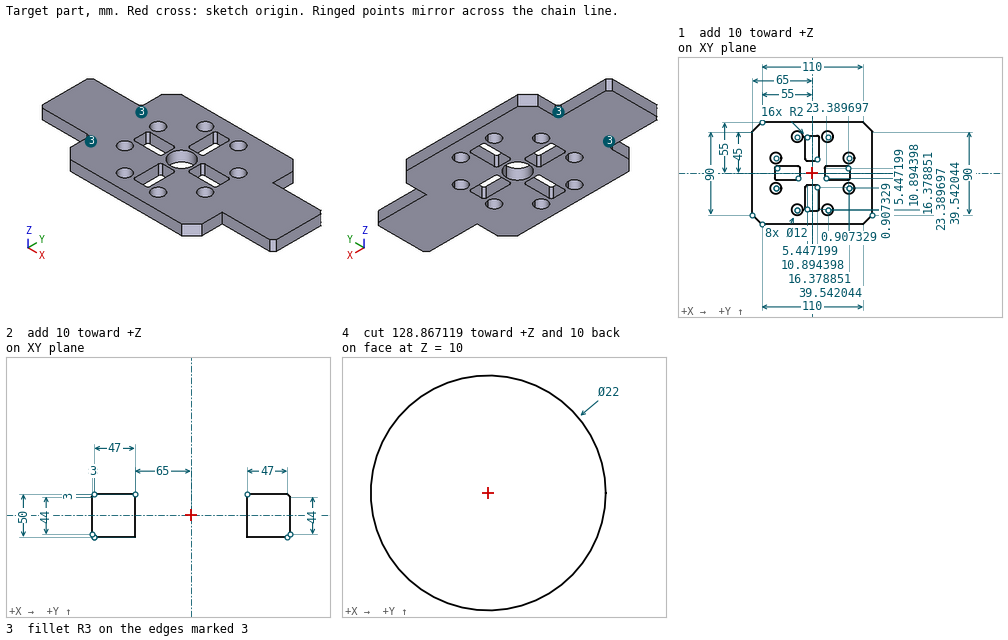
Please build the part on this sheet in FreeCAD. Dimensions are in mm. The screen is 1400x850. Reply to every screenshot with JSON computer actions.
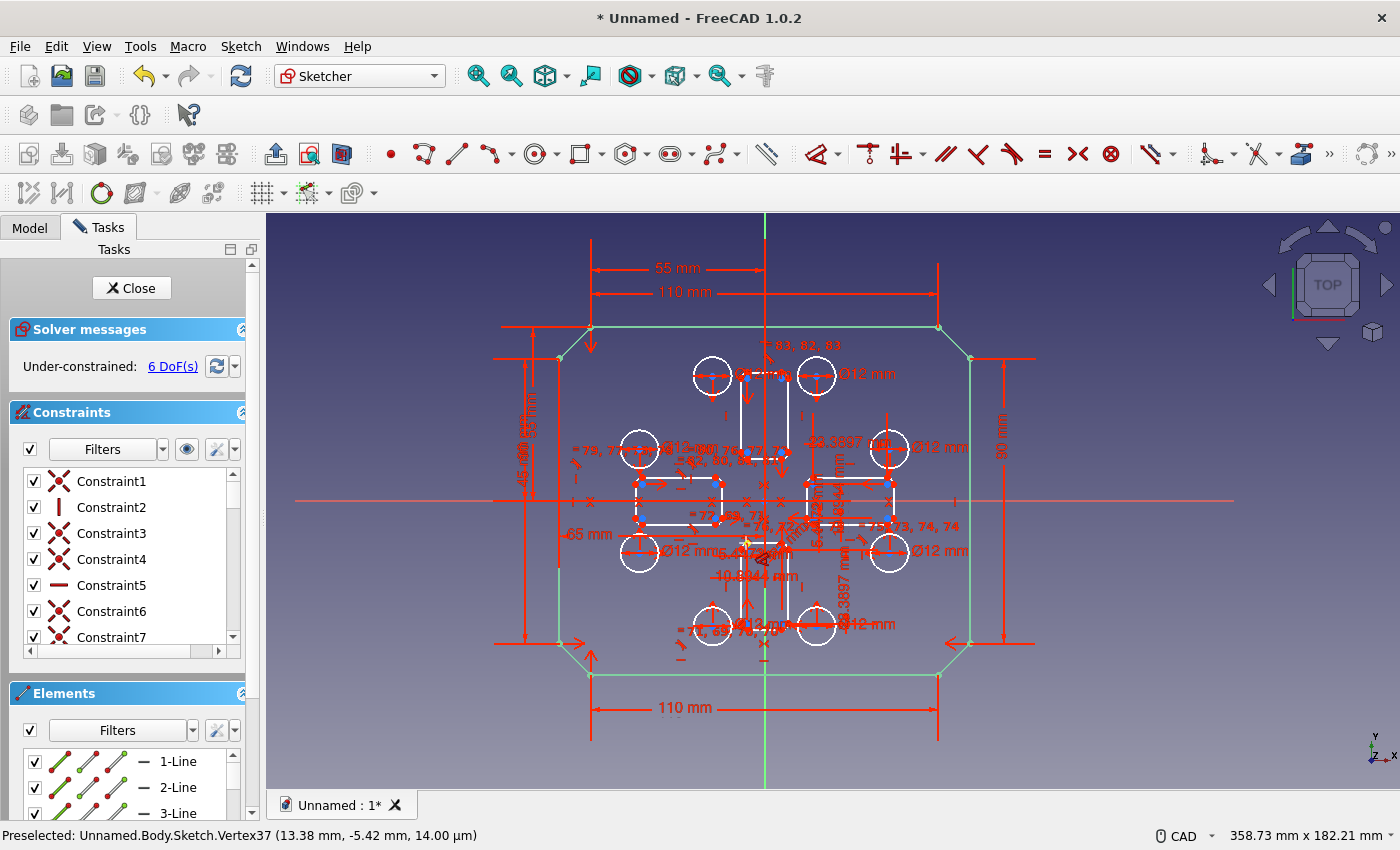
{"action": "left_click", "coordinate": [817, 626]}
{"action": "left_click", "coordinate": [791, 660]}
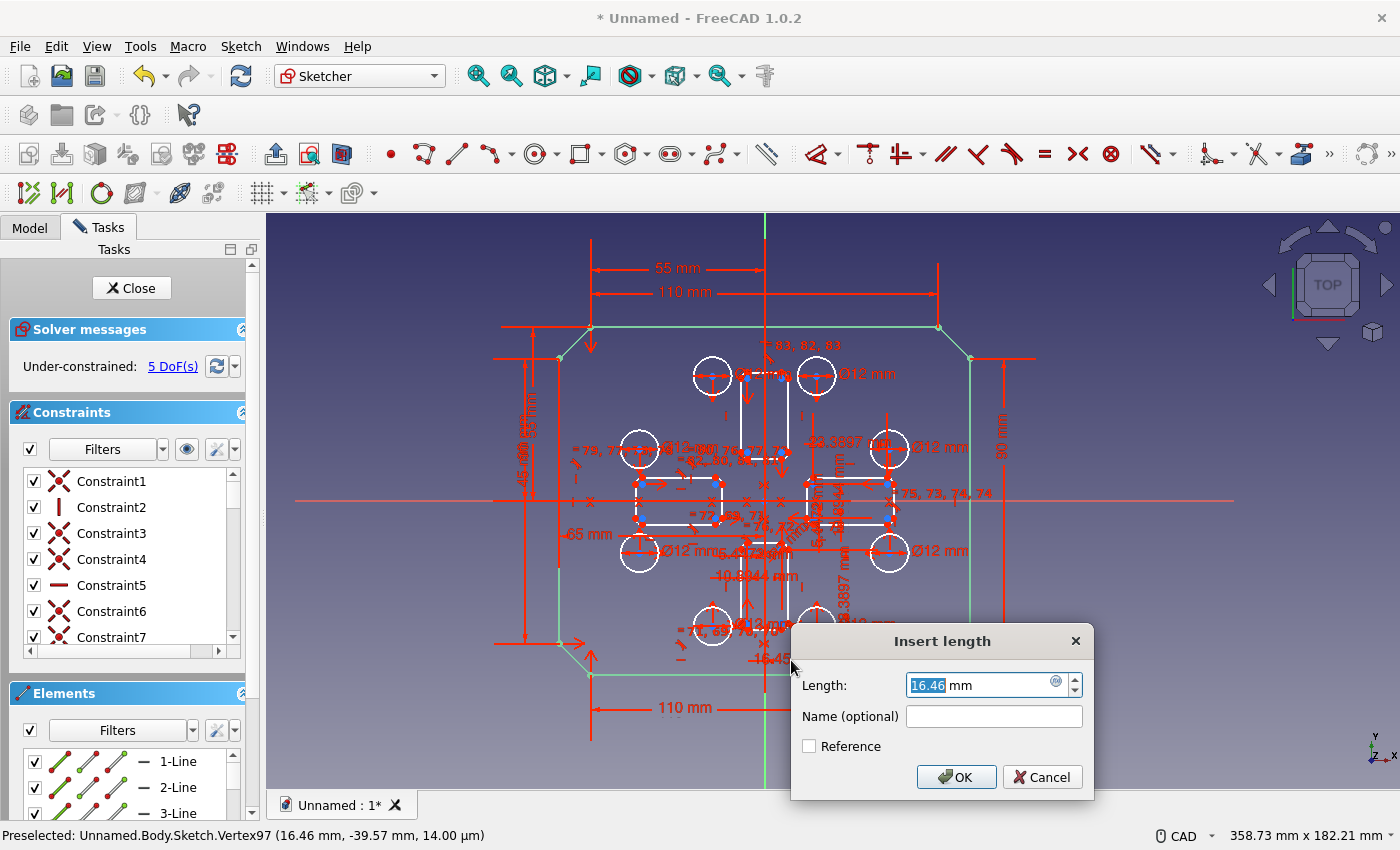
{"action": "type", "text": "16.378851"}
{"action": "key", "text": "Return"}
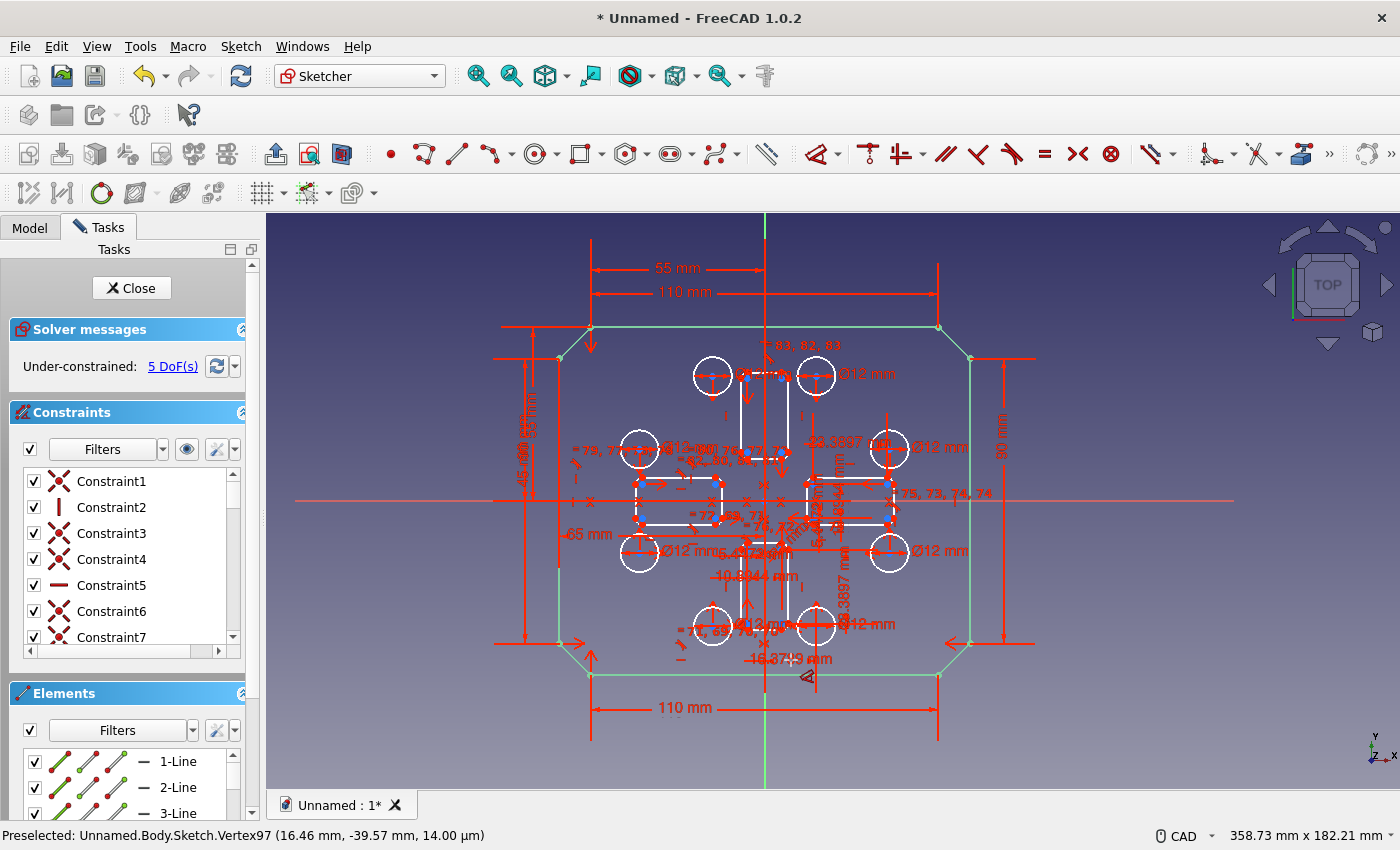
{"action": "left_click", "coordinate": [816, 626]}
{"action": "left_click", "coordinate": [850, 564]}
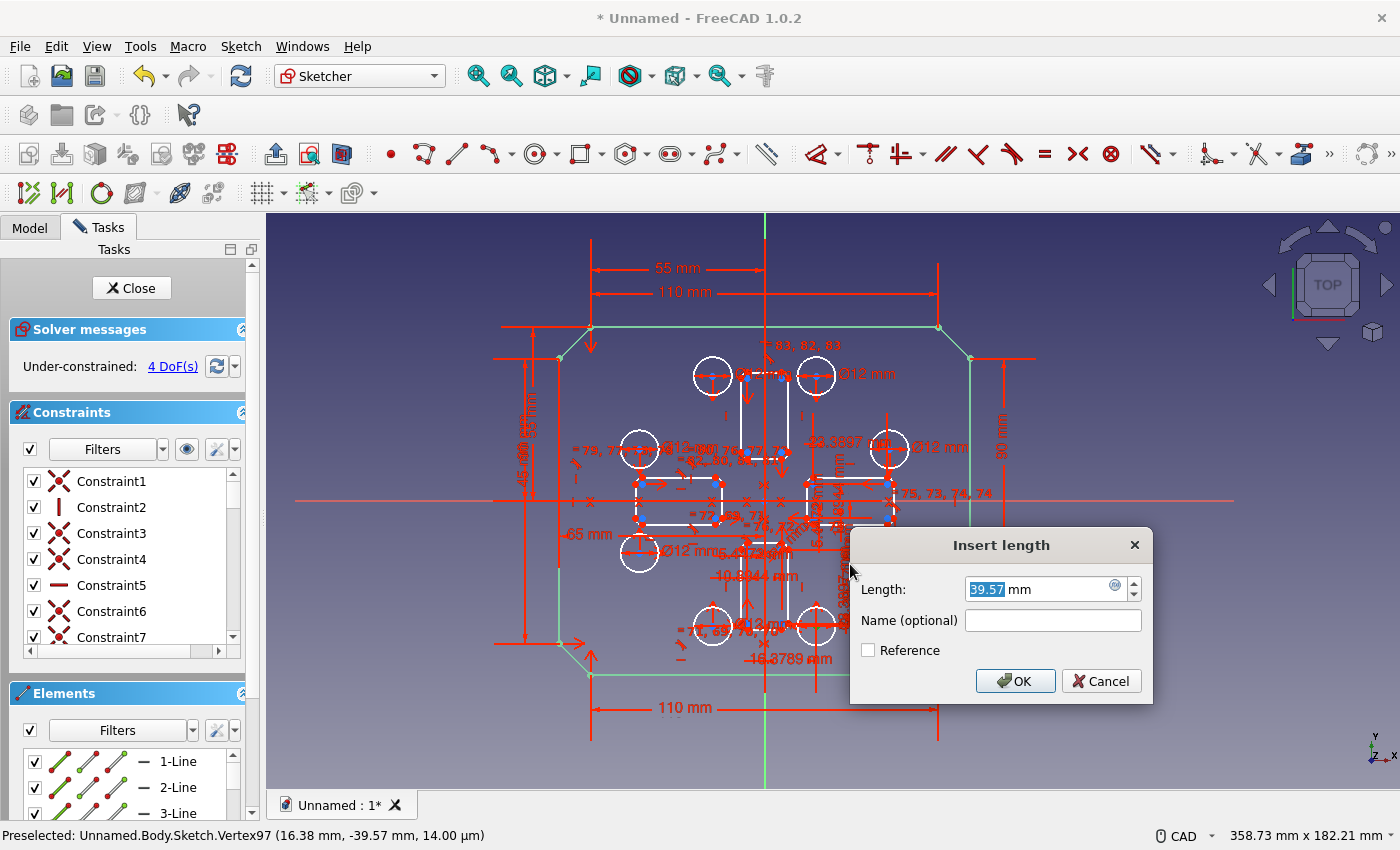
{"action": "type", "text": "39.542044"}
{"action": "key", "text": "Return"}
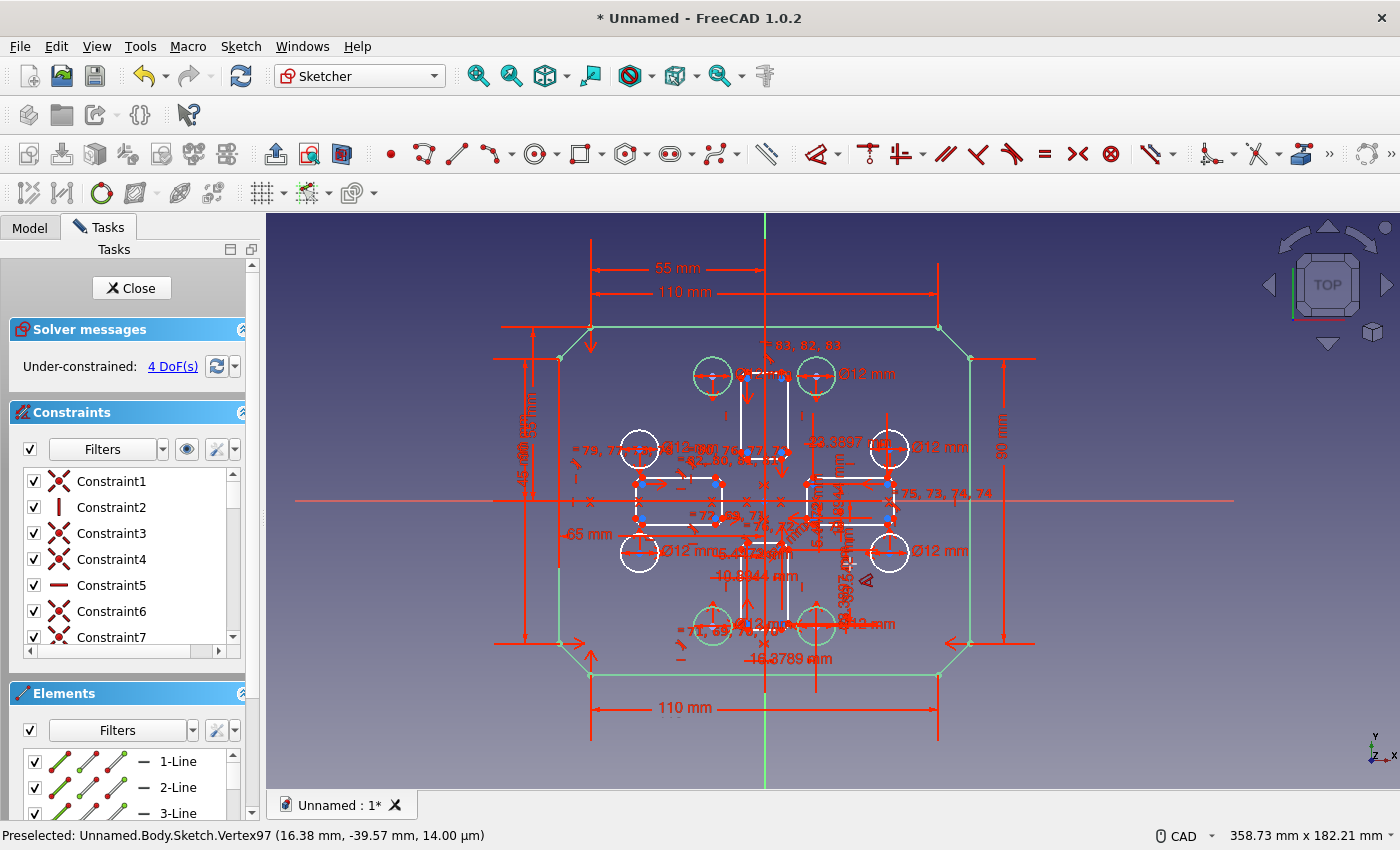
{"action": "left_click", "coordinate": [890, 553]}
{"action": "left_click", "coordinate": [798, 467]}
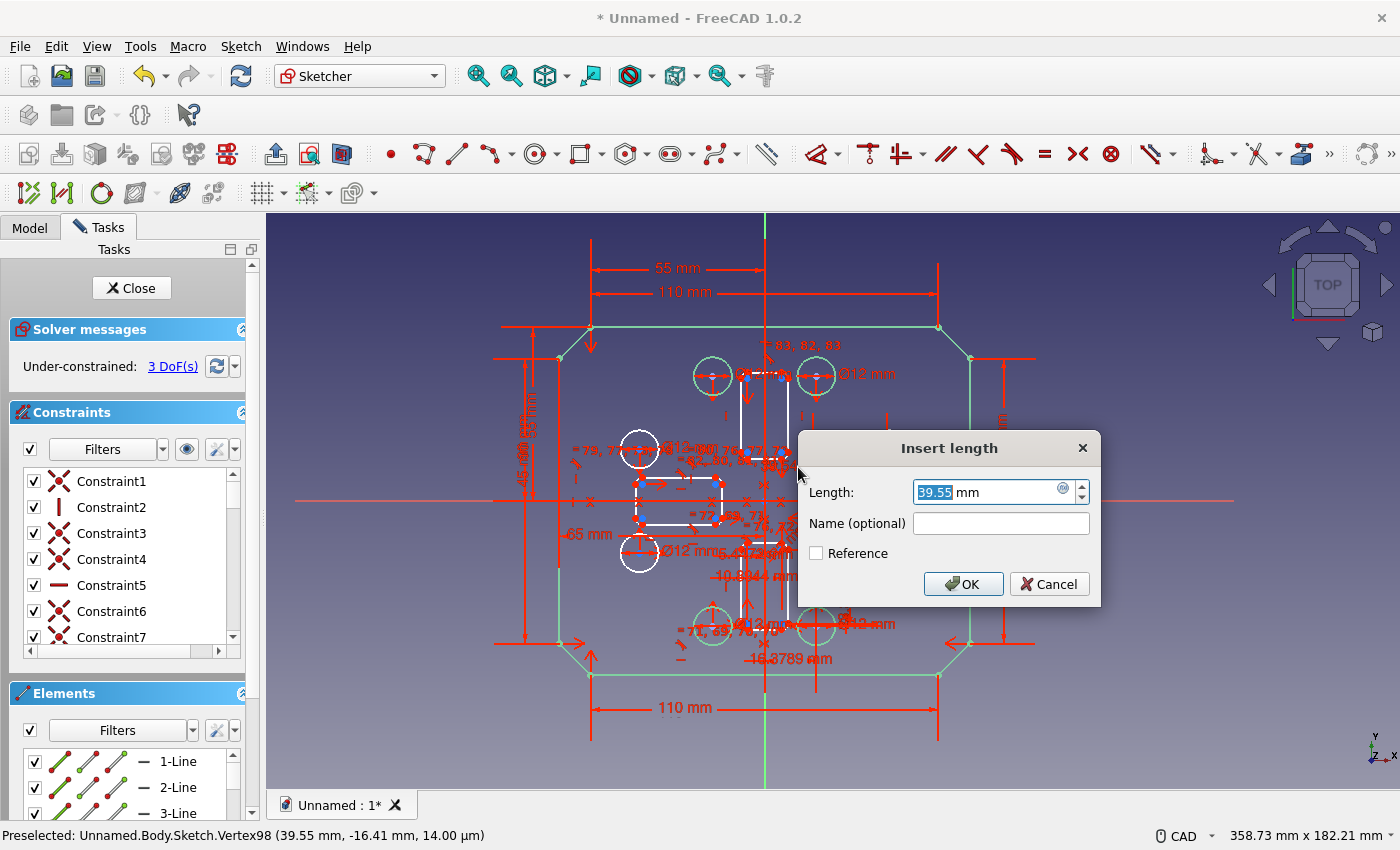
{"action": "type", "text": "39.542044"}
{"action": "key", "text": "Return"}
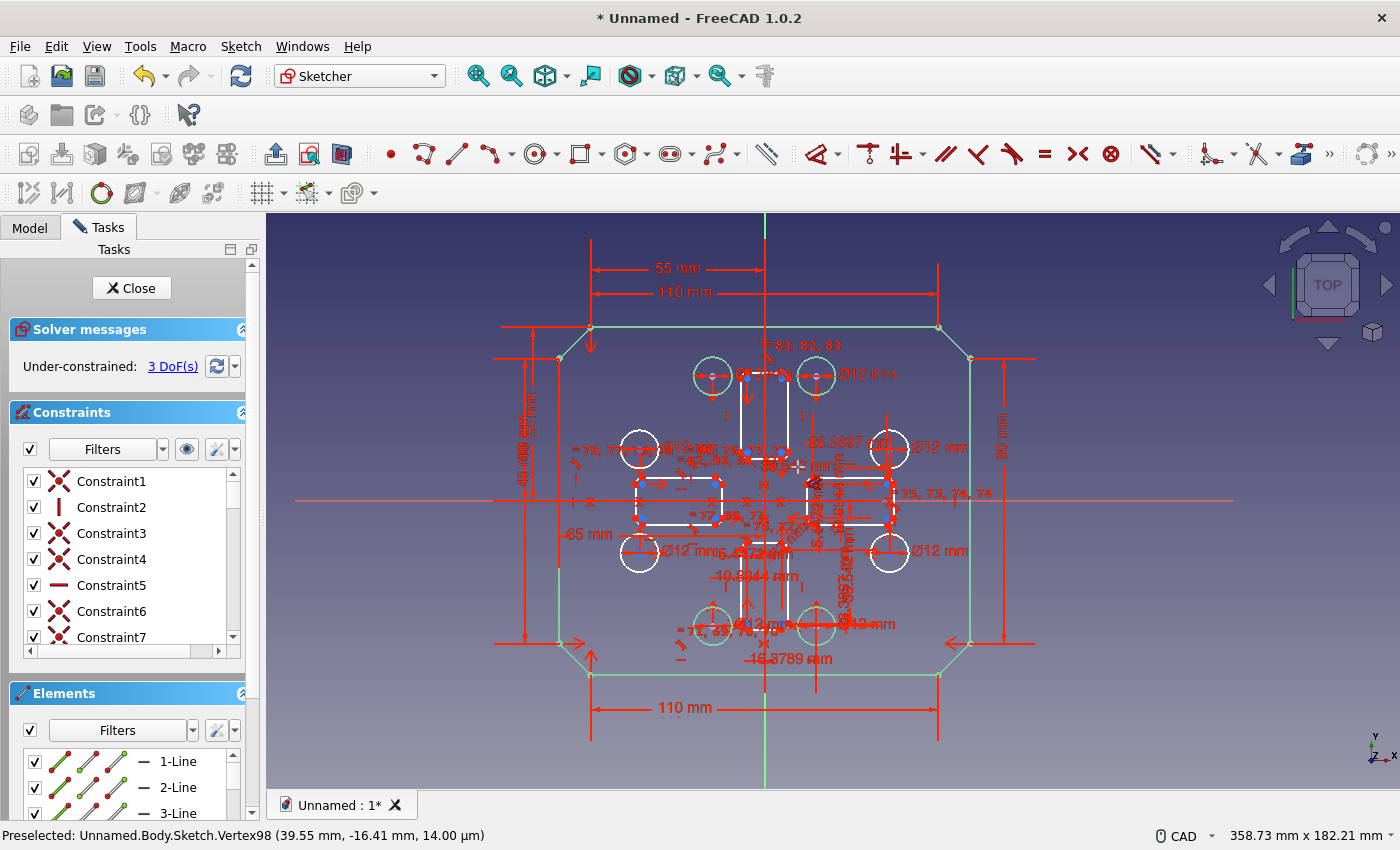
{"action": "left_click", "coordinate": [890, 553]}
{"action": "left_click", "coordinate": [924, 527]}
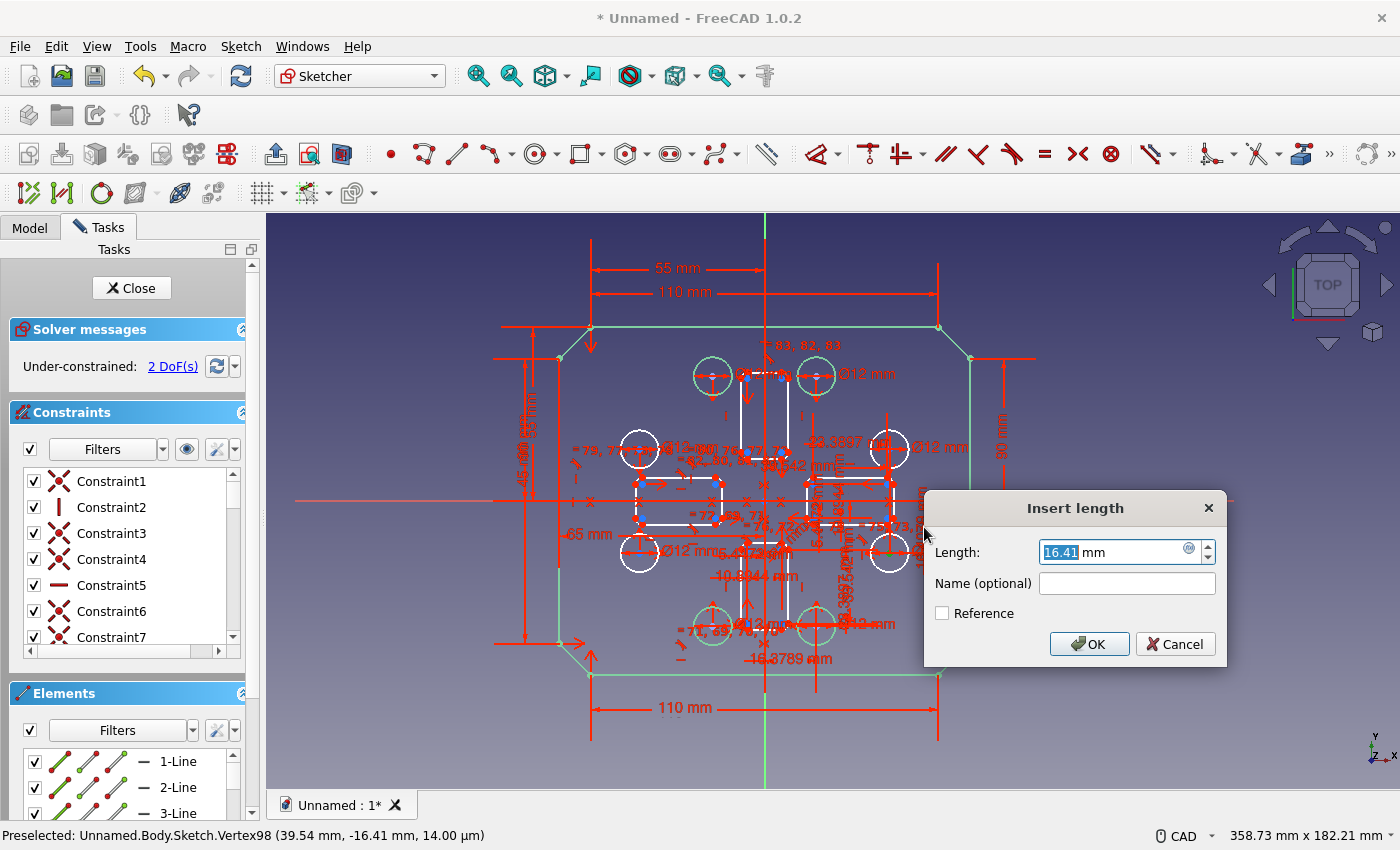
{"action": "type", "text": "16.378851"}
{"action": "key", "text": "Return"}